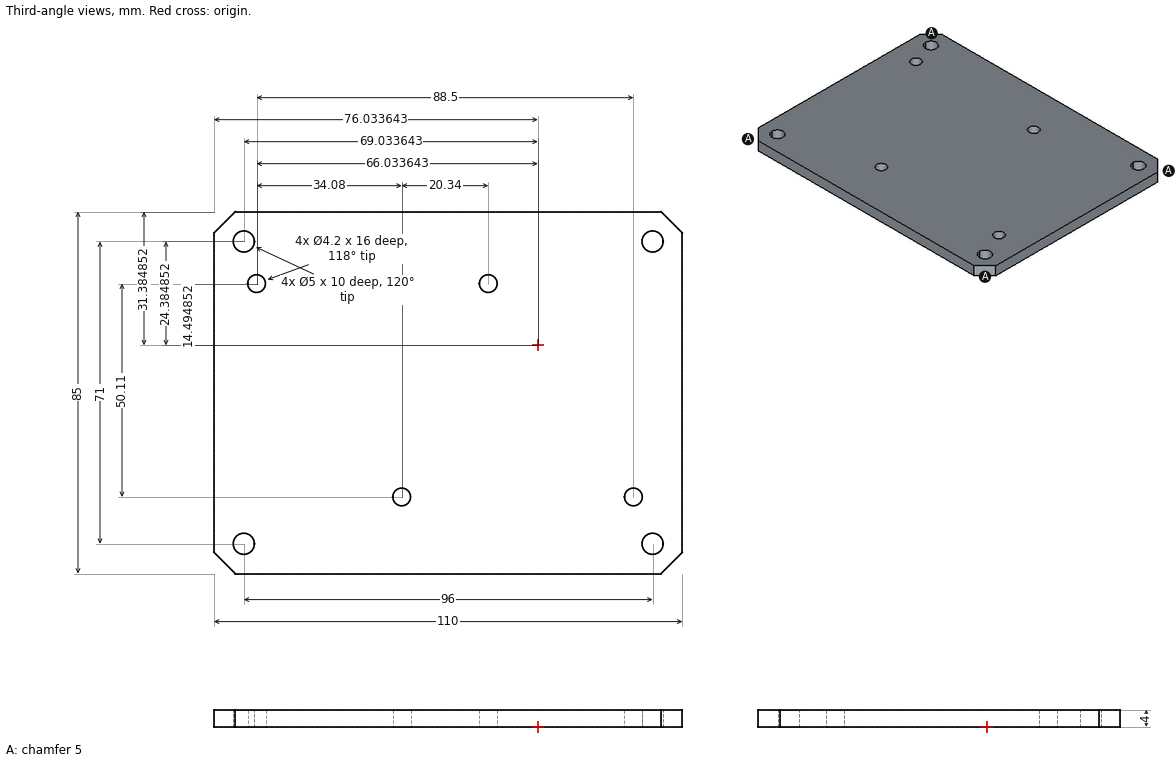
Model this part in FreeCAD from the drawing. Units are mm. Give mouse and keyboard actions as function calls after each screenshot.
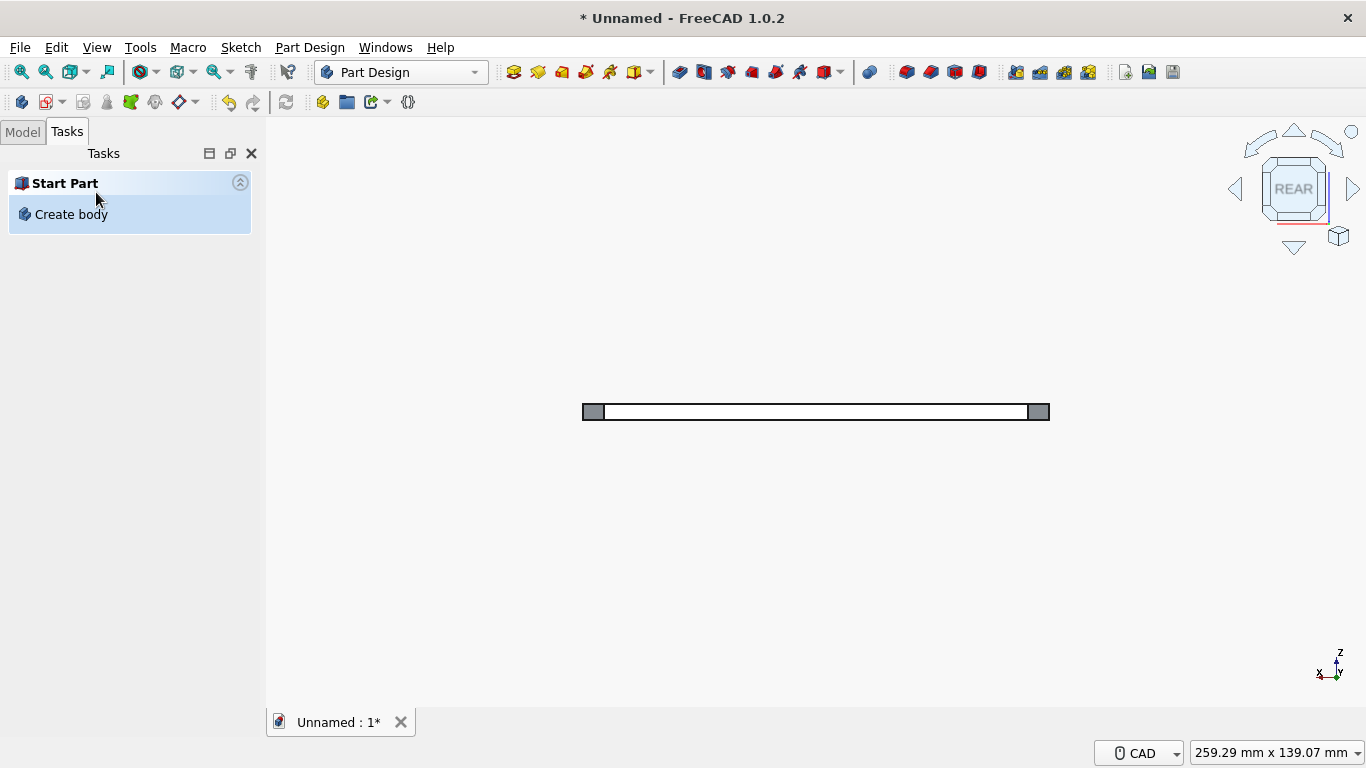
click(22, 72)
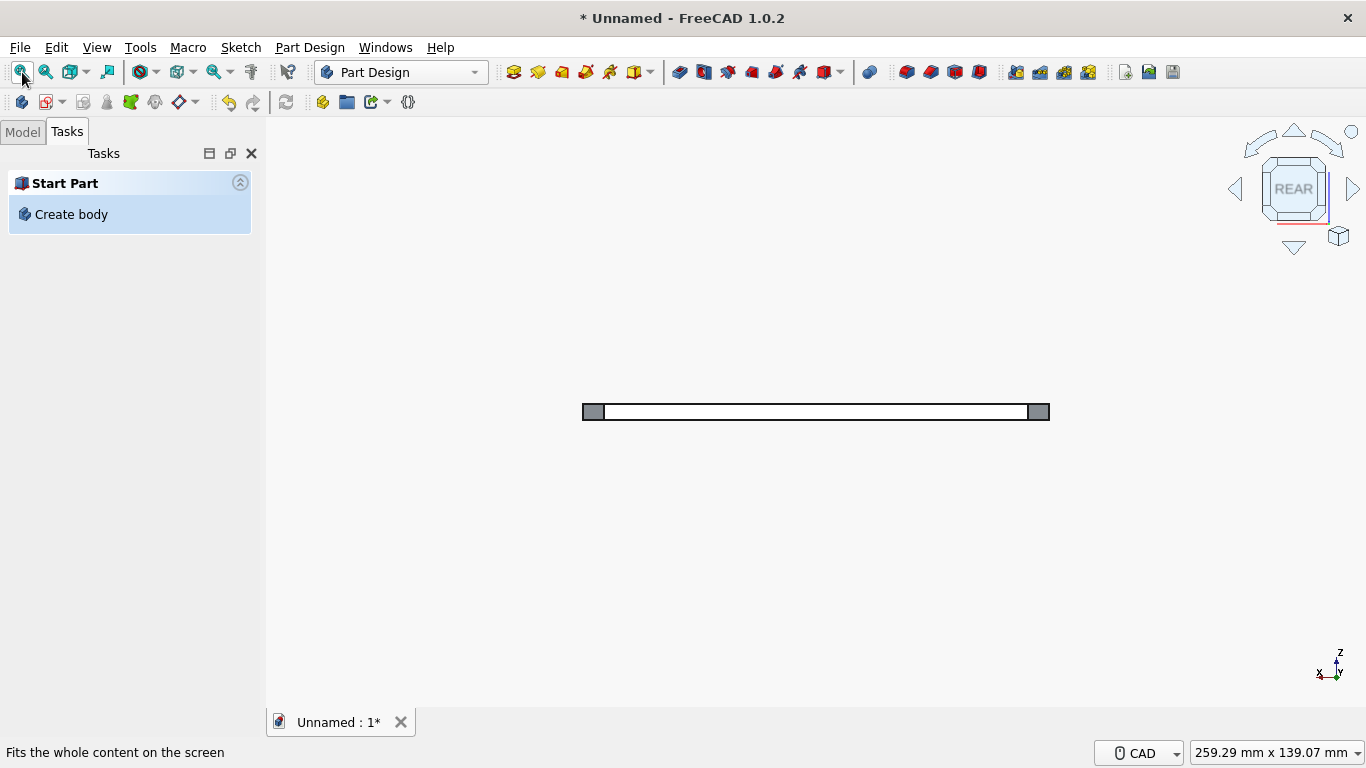
key(5)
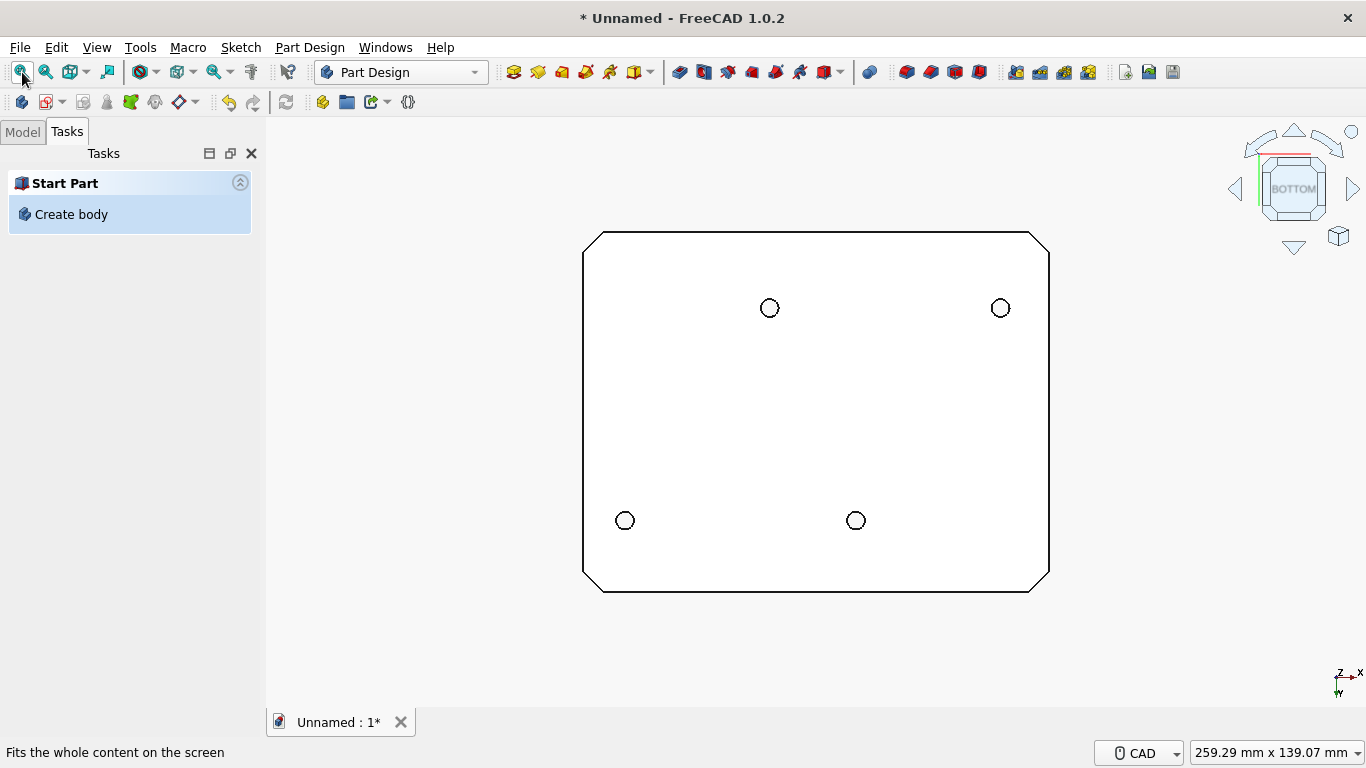
click(883, 359)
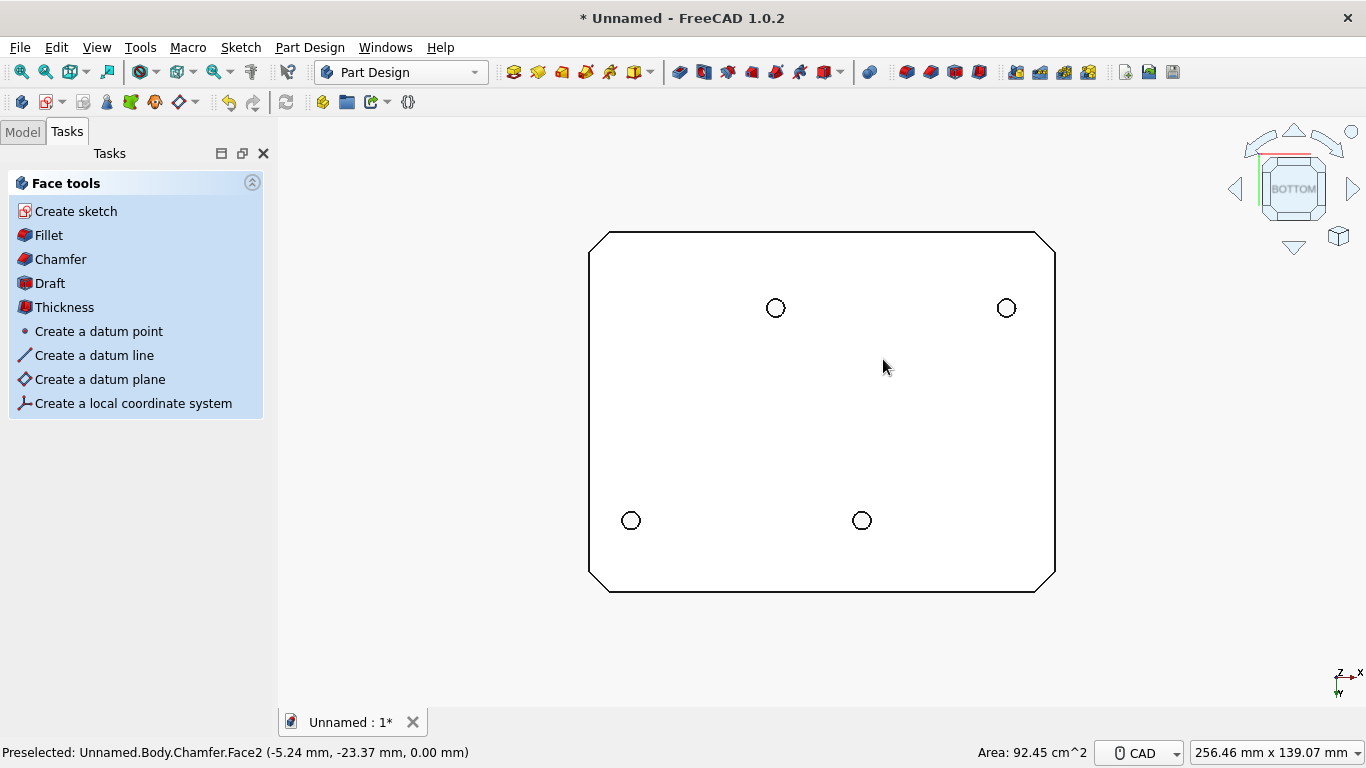
click(46, 102)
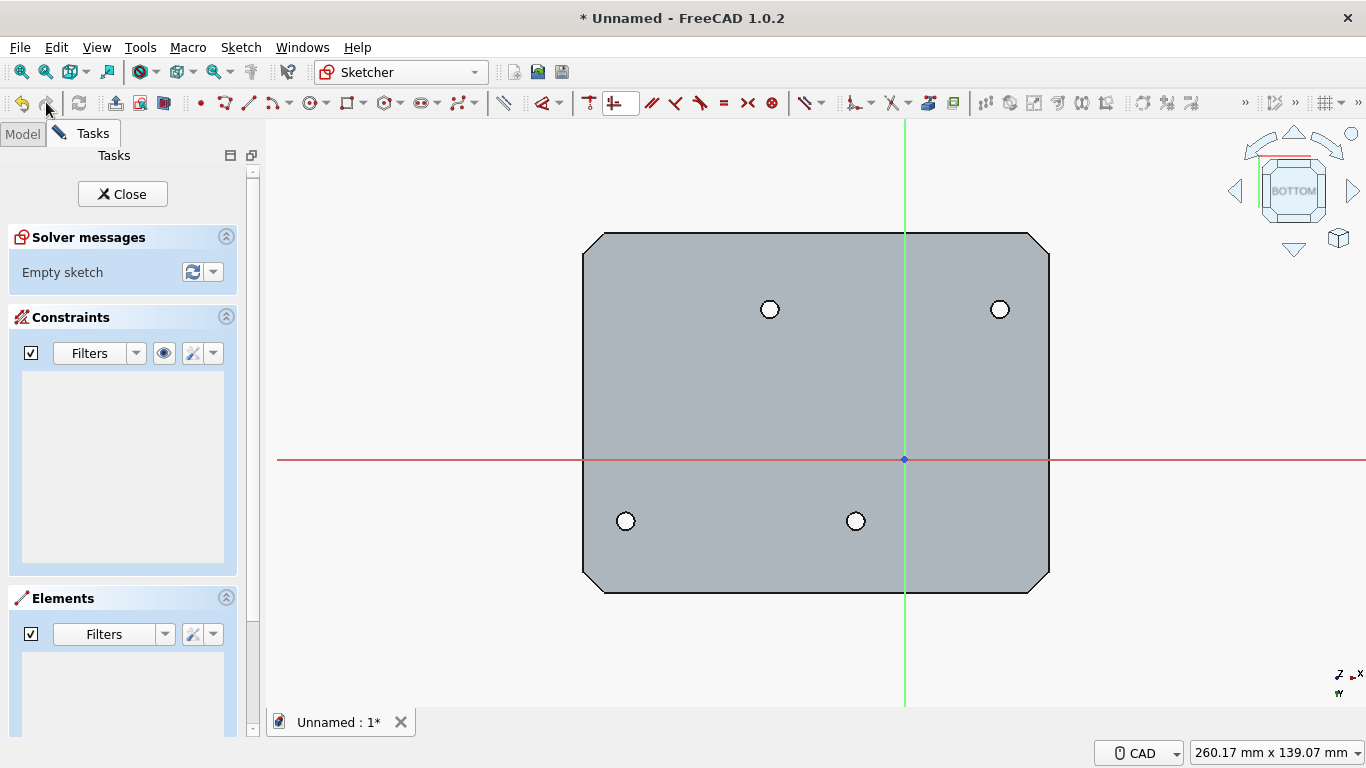
click(310, 104)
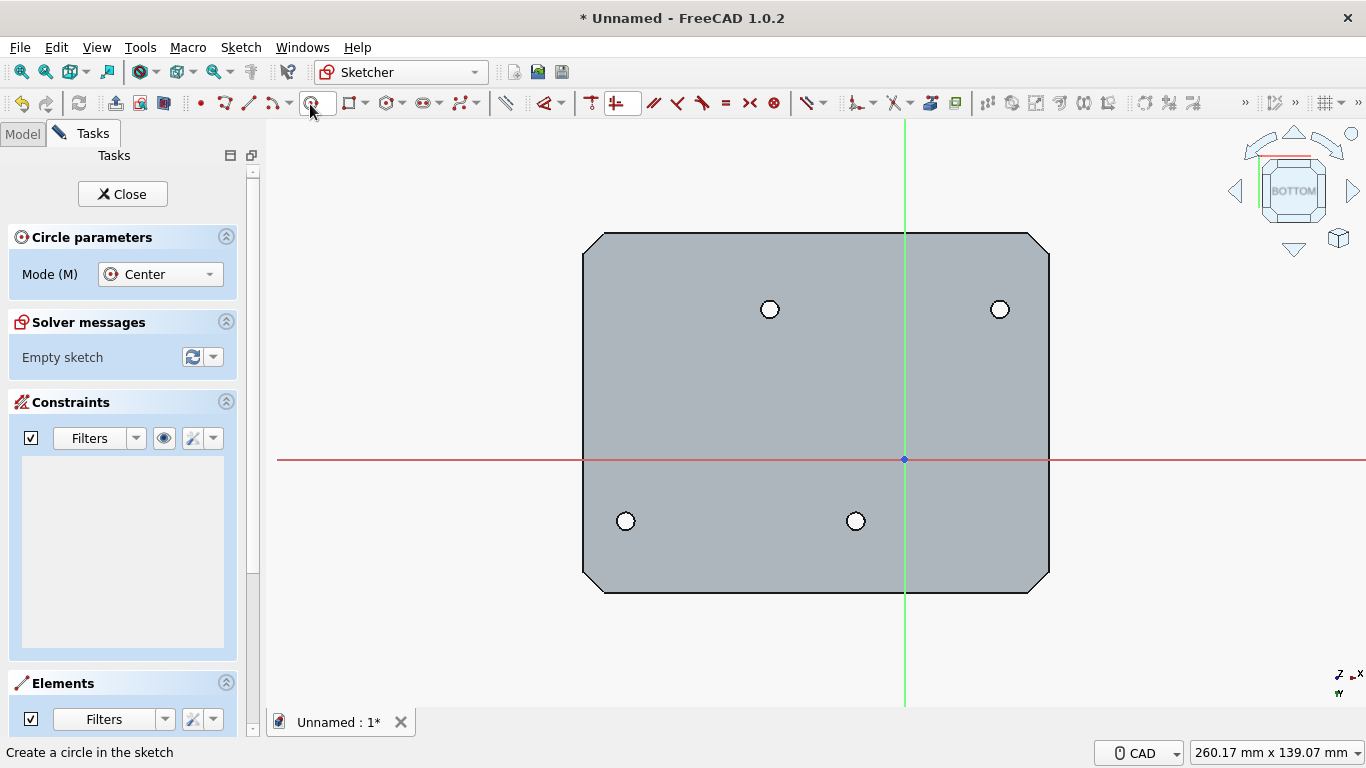
scroll(613, 563, up, 4)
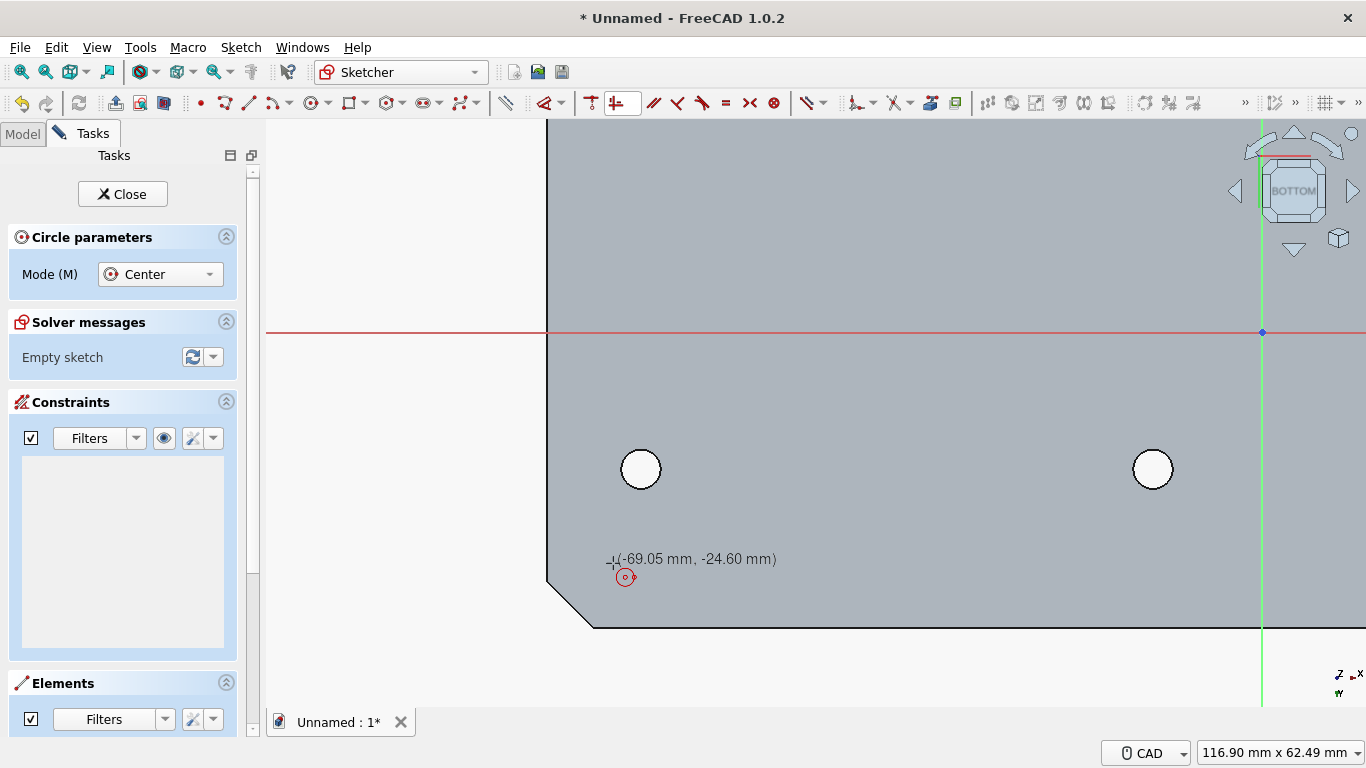
click(613, 562)
click(629, 546)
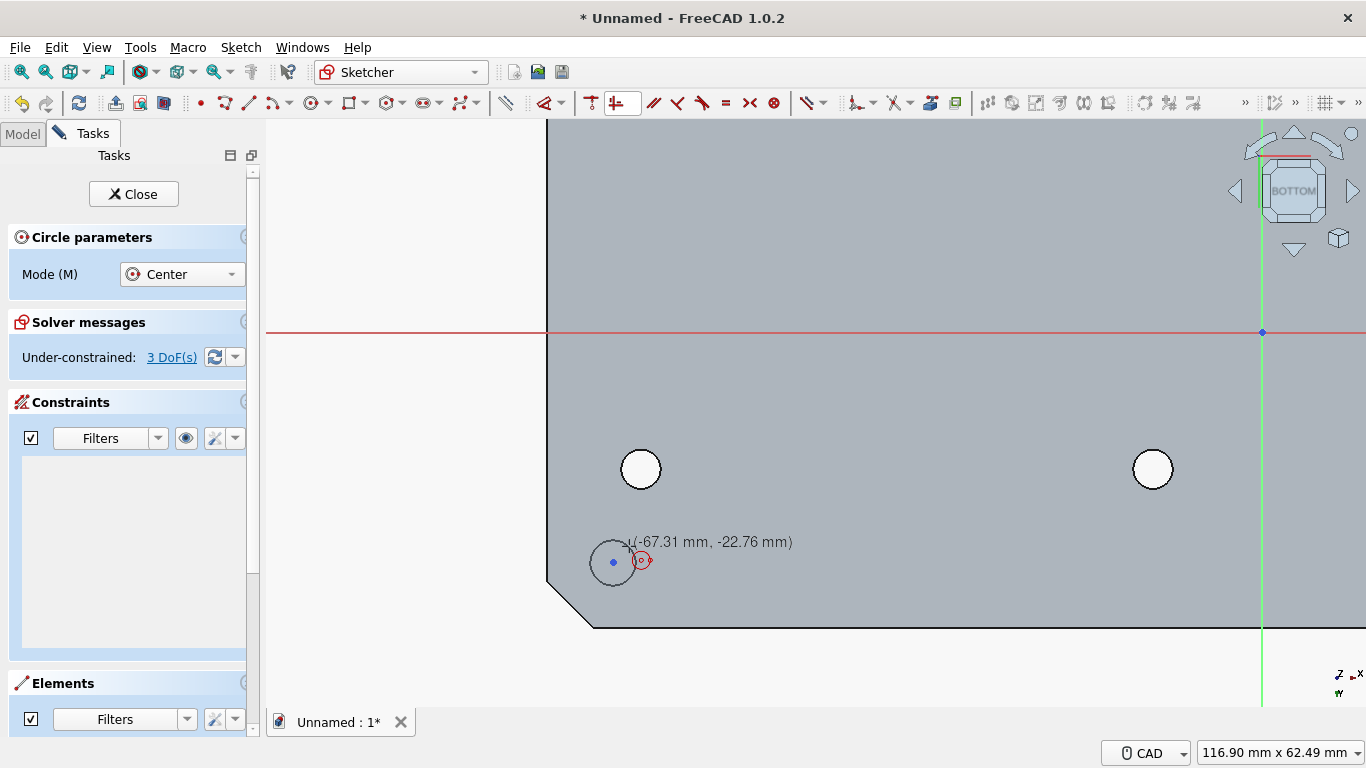
scroll(362, 638, down, 3)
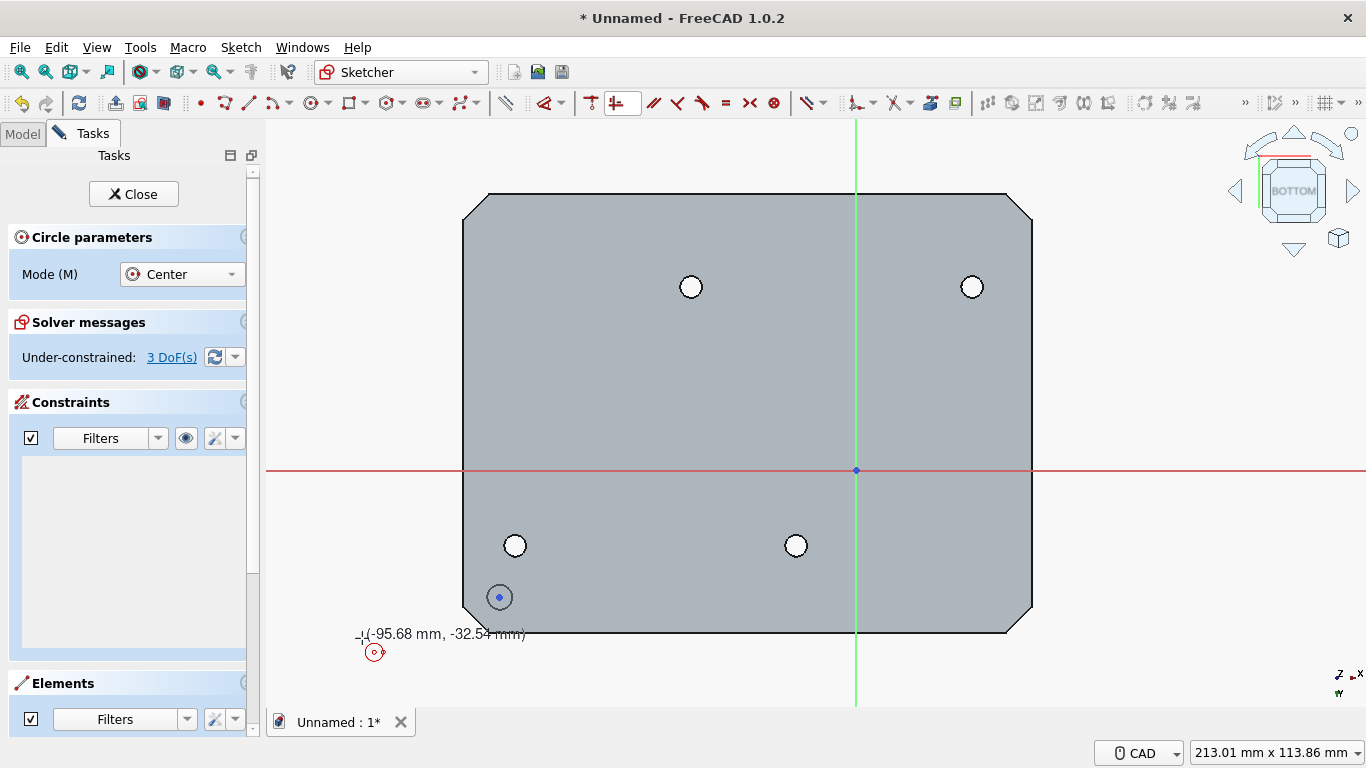
scroll(500, 230, up, 3)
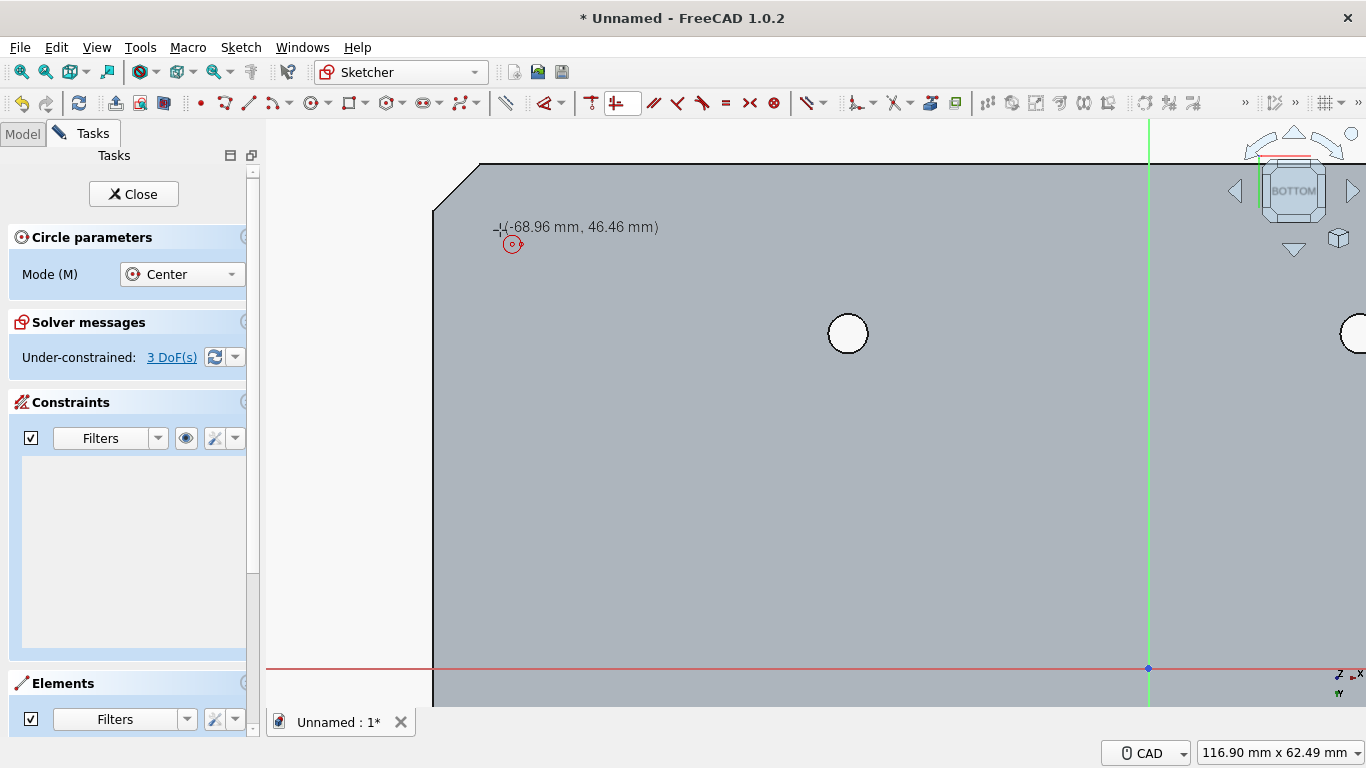
click(499, 230)
click(516, 214)